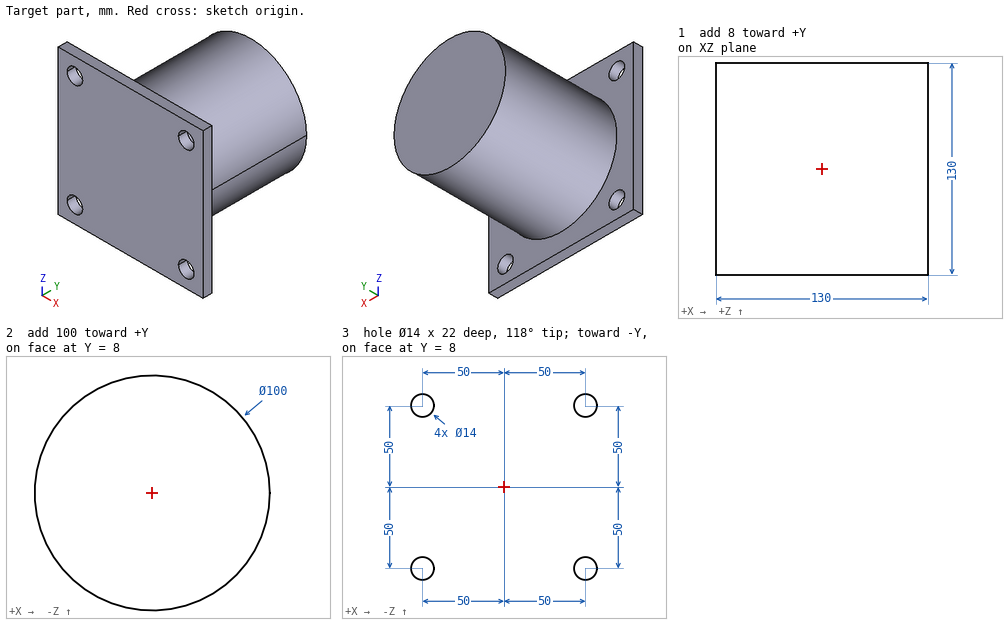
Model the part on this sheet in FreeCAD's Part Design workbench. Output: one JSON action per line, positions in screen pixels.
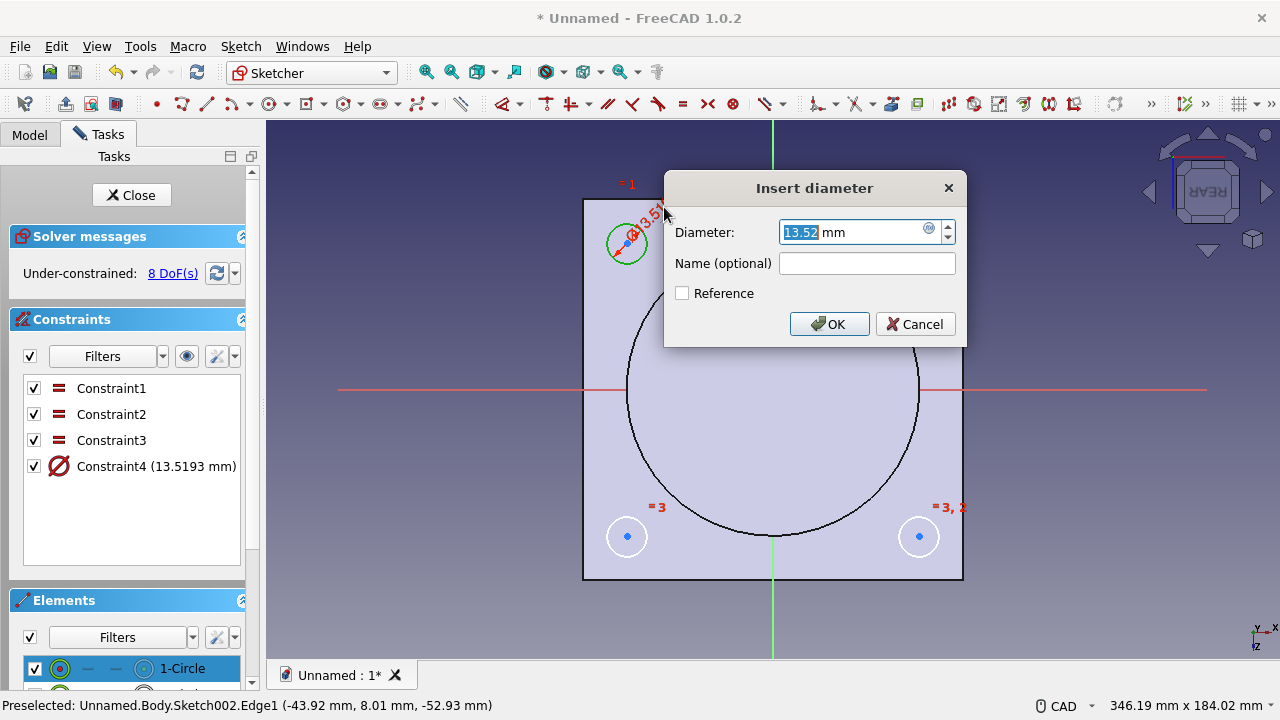
{"action": "type", "text": "14"}
{"action": "key", "text": "Return"}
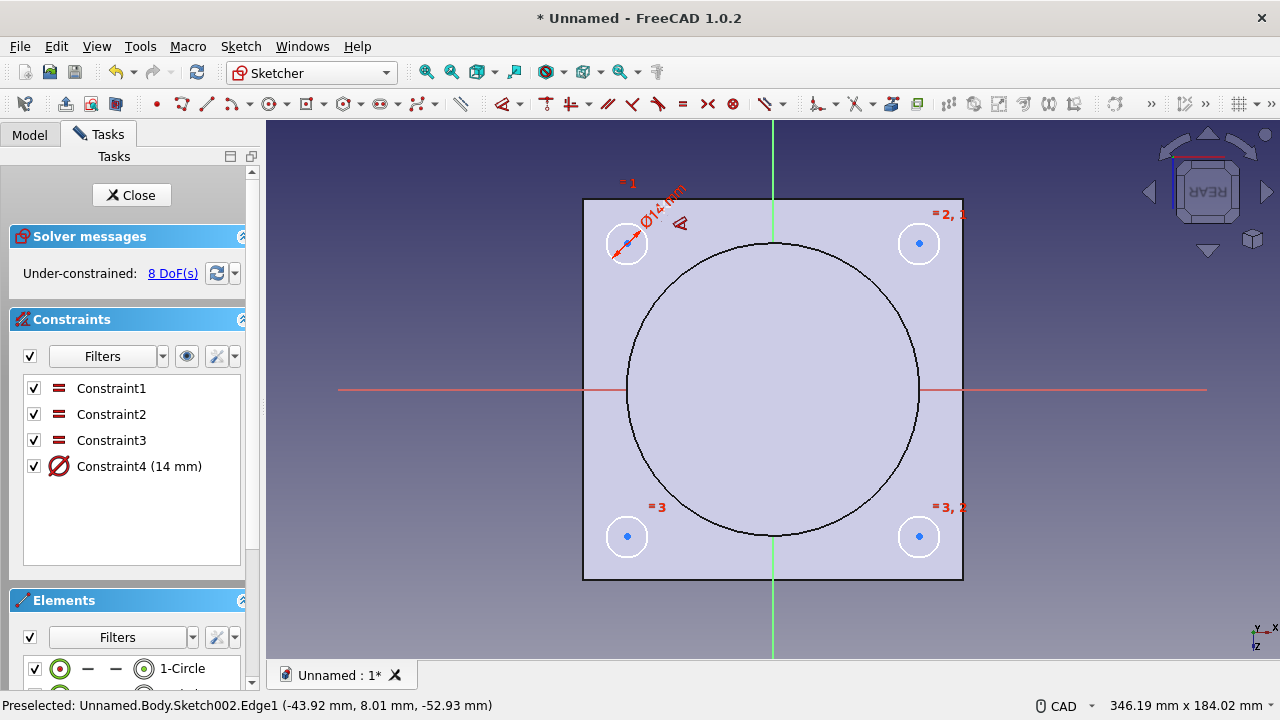
{"action": "left_click", "coordinate": [627, 244]}
{"action": "left_click", "coordinate": [751, 210]}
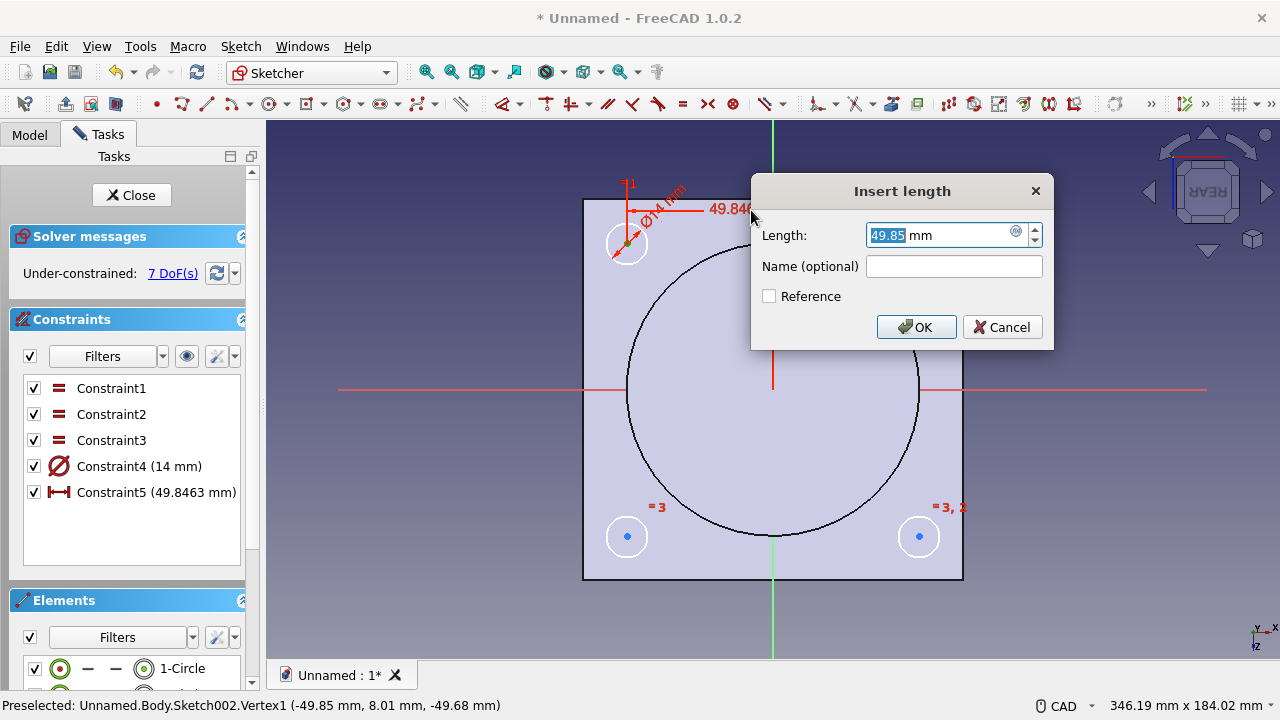
{"action": "type", "text": "50"}
{"action": "key", "text": "Return"}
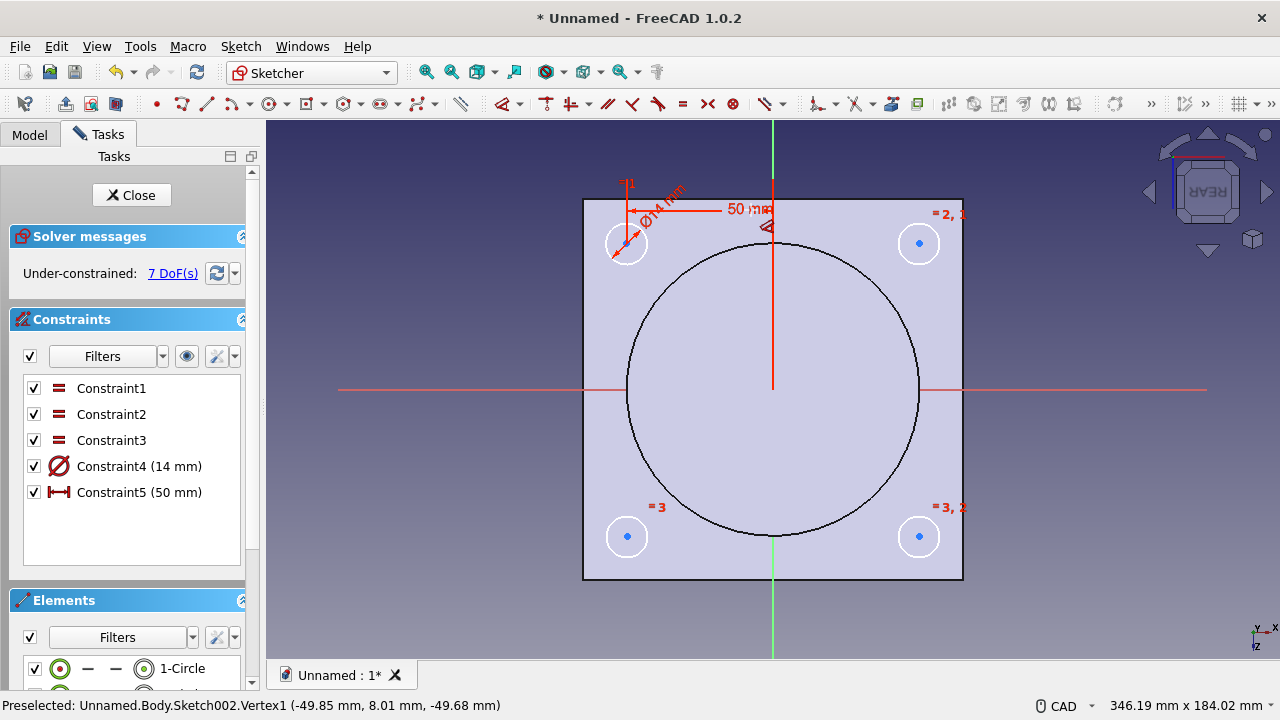
{"action": "left_click", "coordinate": [627, 244]}
{"action": "left_click", "coordinate": [593, 317]}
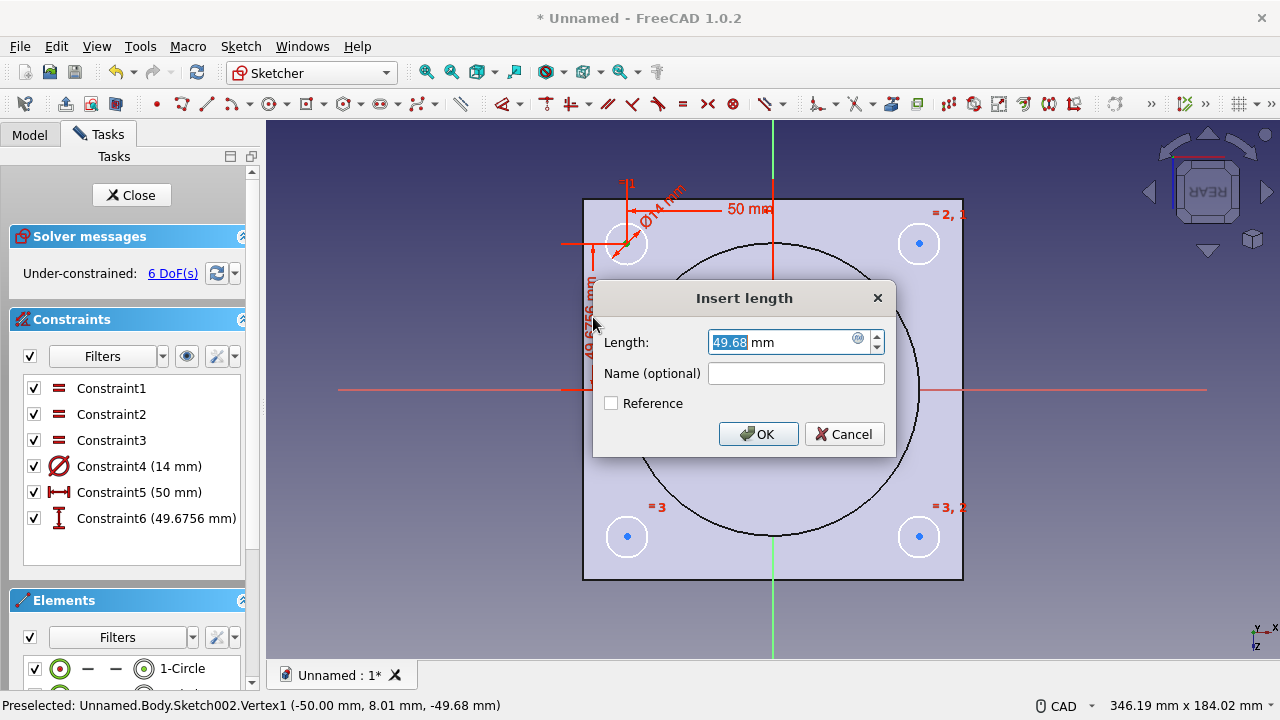
{"action": "type", "text": "50"}
{"action": "key", "text": "Return"}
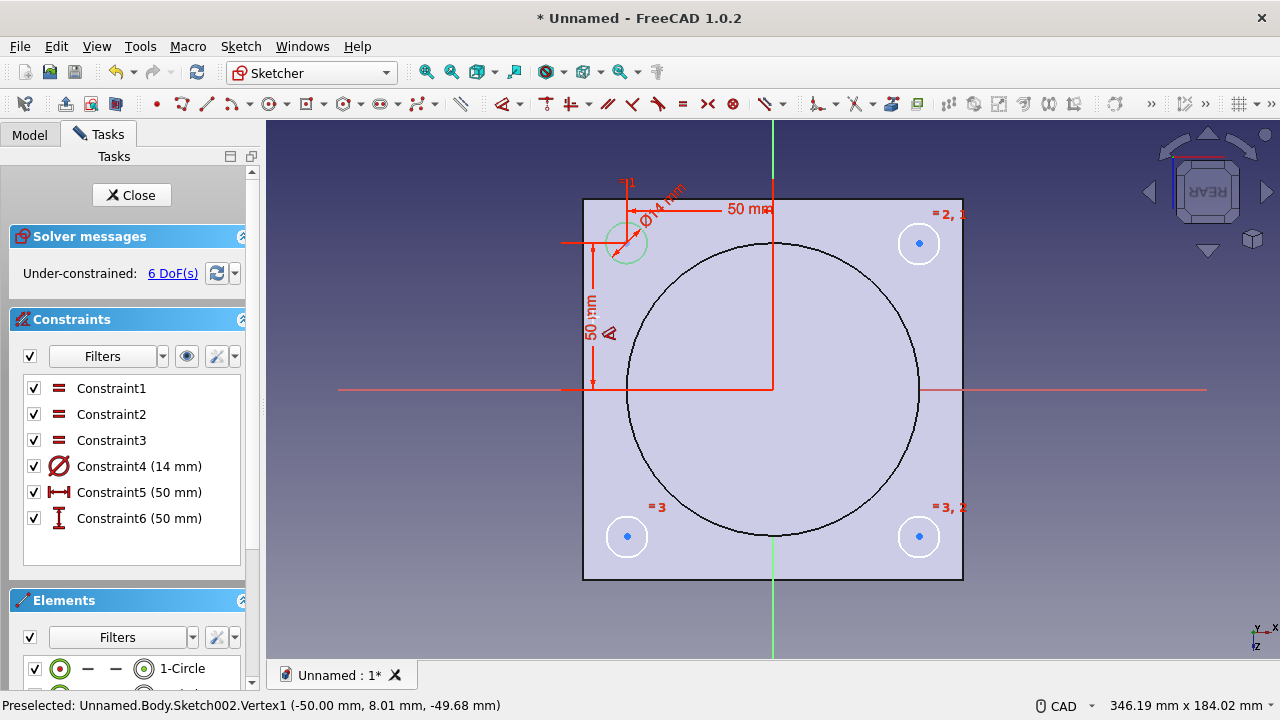
{"action": "left_click", "coordinate": [919, 244]}
{"action": "left_click", "coordinate": [846, 210]}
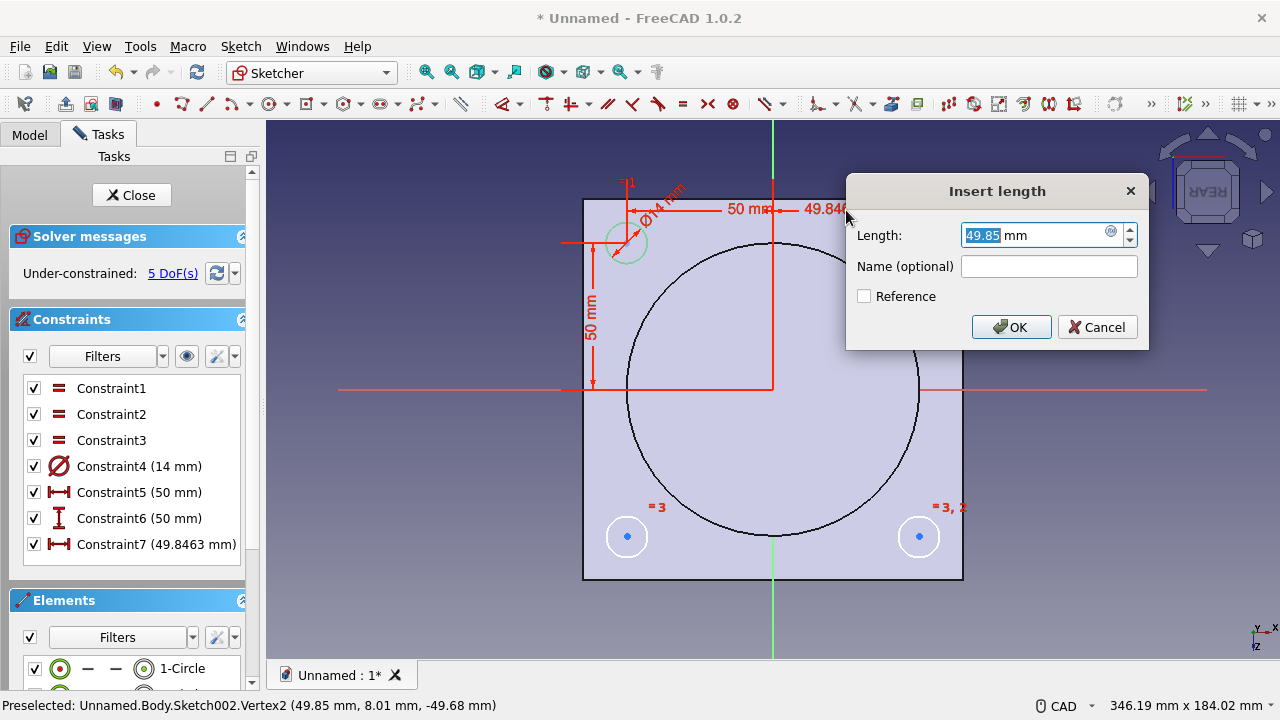
{"action": "type", "text": "50"}
{"action": "key", "text": "Return"}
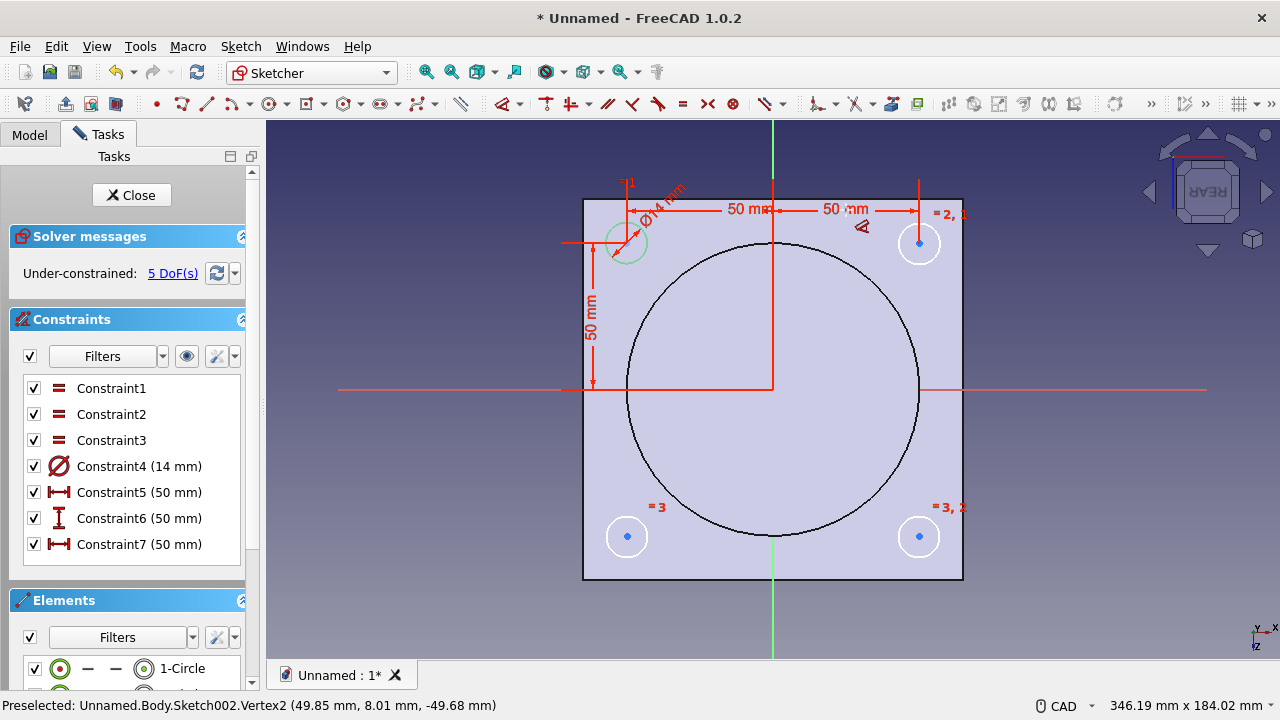
{"action": "left_click", "coordinate": [919, 244]}
{"action": "left_click", "coordinate": [953, 317]}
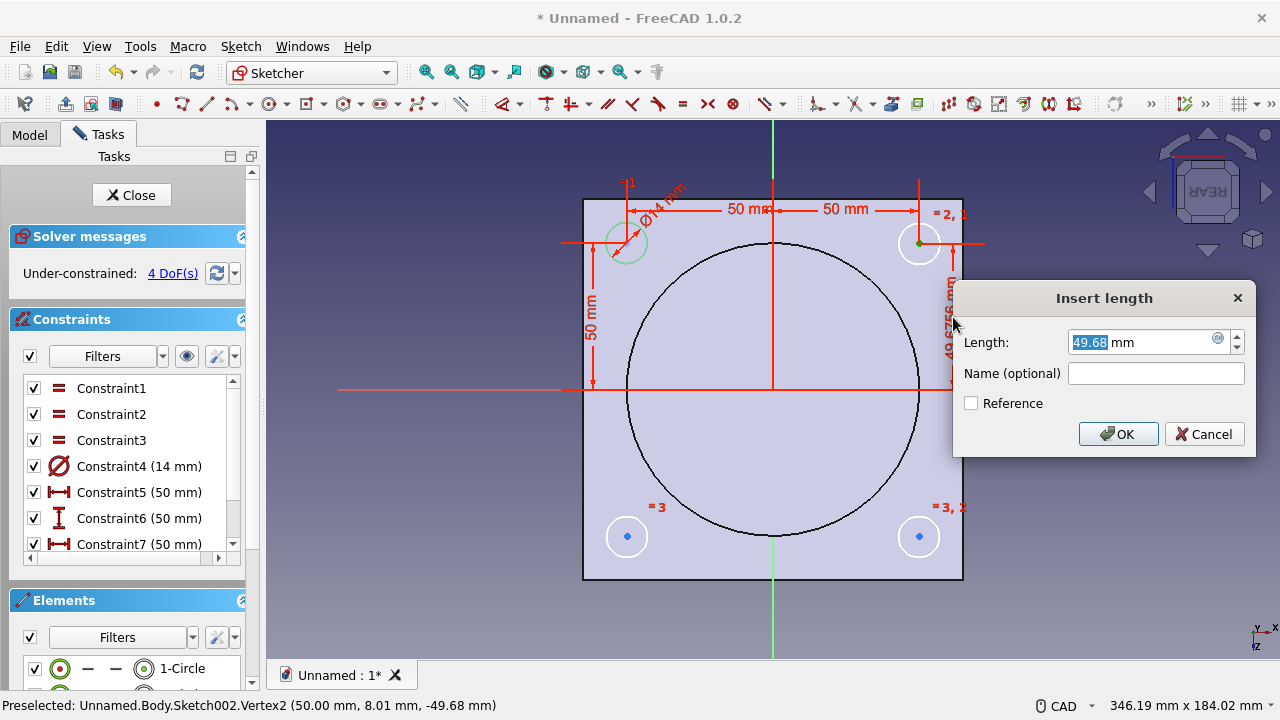
{"action": "type", "text": "50"}
{"action": "key", "text": "Return"}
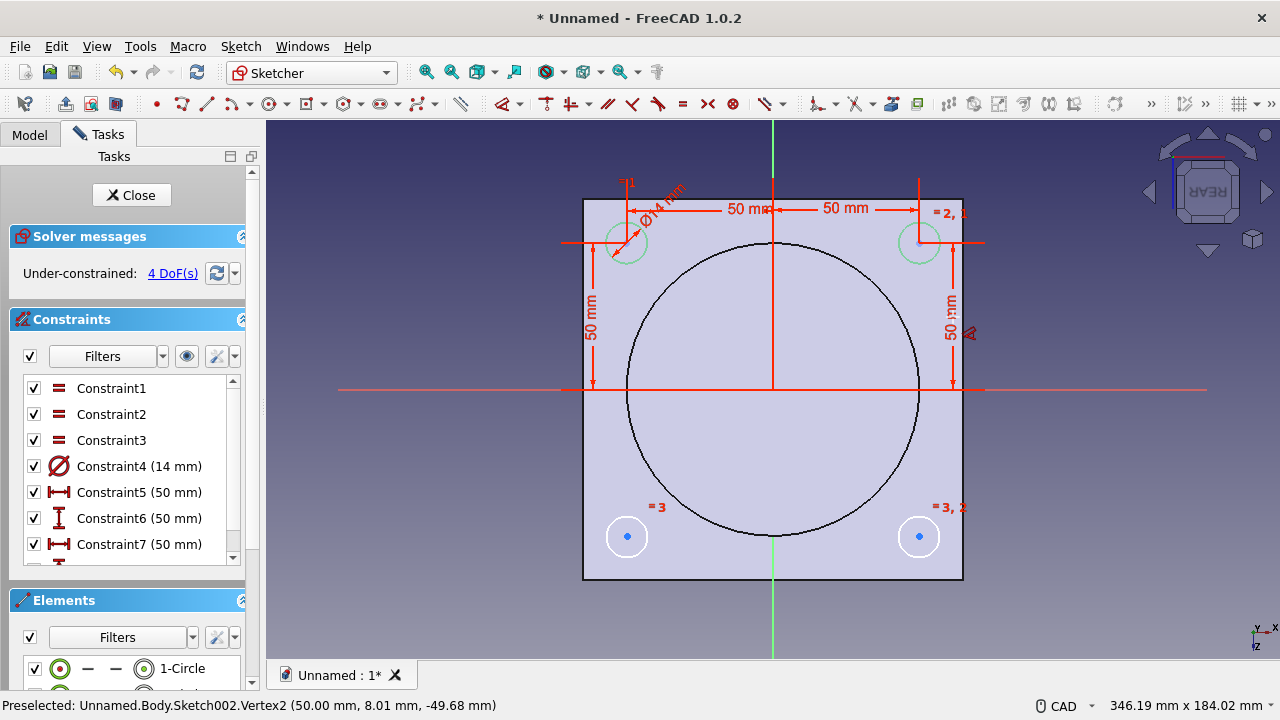
{"action": "left_click", "coordinate": [919, 537]}
{"action": "left_click", "coordinate": [846, 571]}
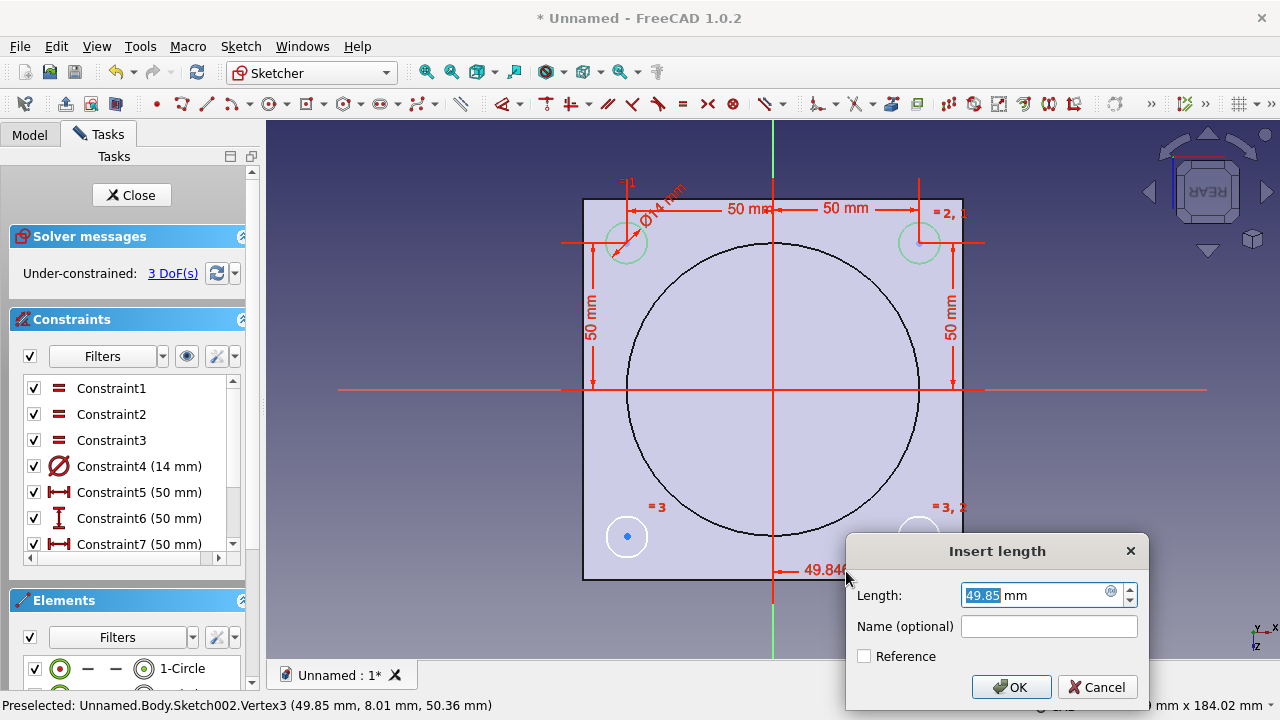
{"action": "type", "text": "50"}
{"action": "key", "text": "Return"}